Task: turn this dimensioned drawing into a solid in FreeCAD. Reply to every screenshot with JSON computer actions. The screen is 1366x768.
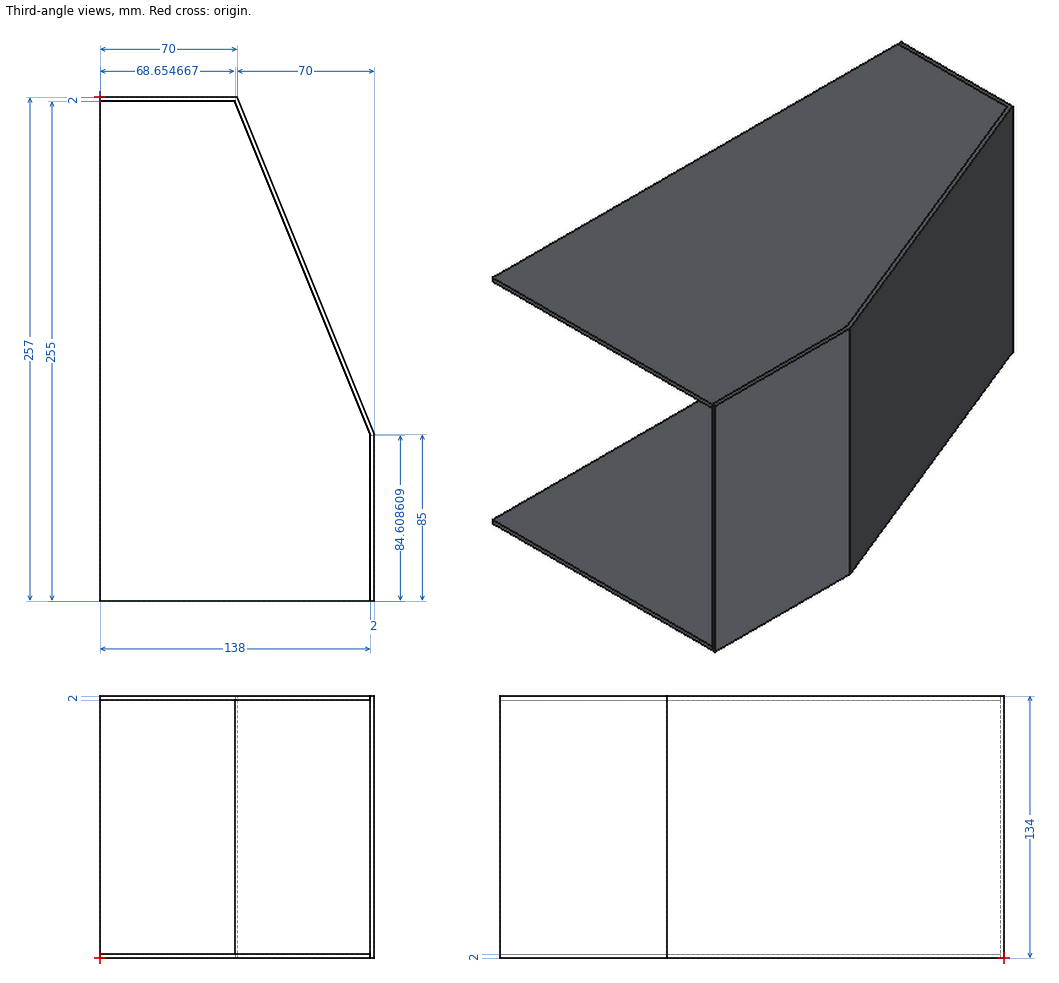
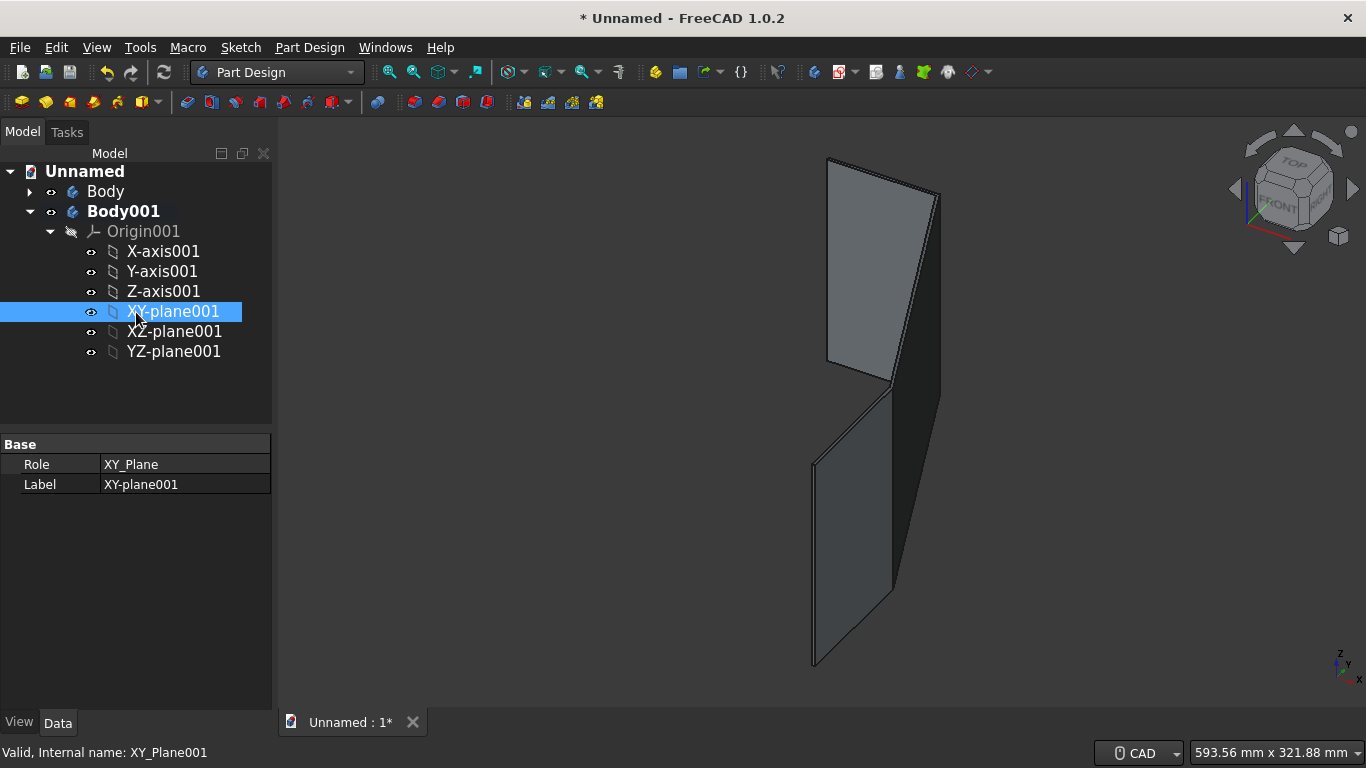
{"action": "left_click", "coordinate": [972, 72]}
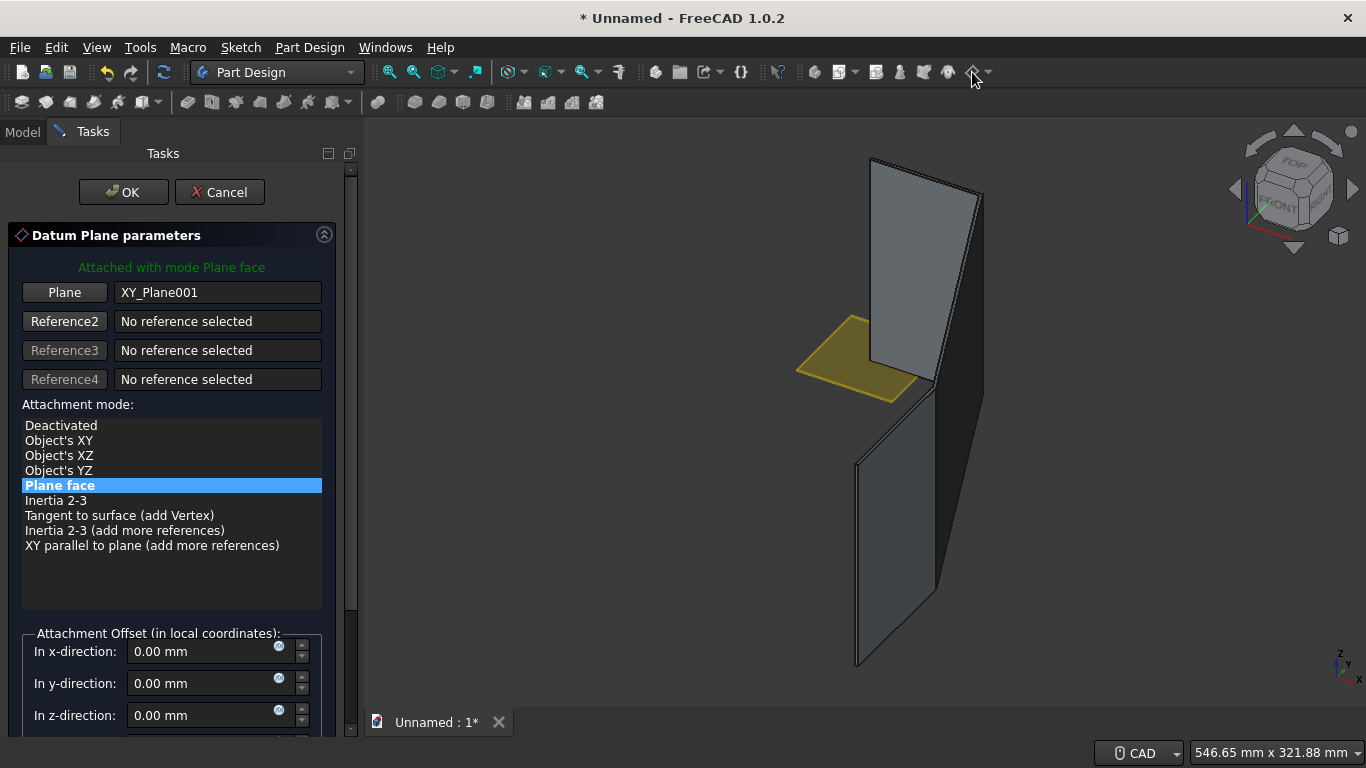
{"action": "triple_click", "coordinate": [210, 715]}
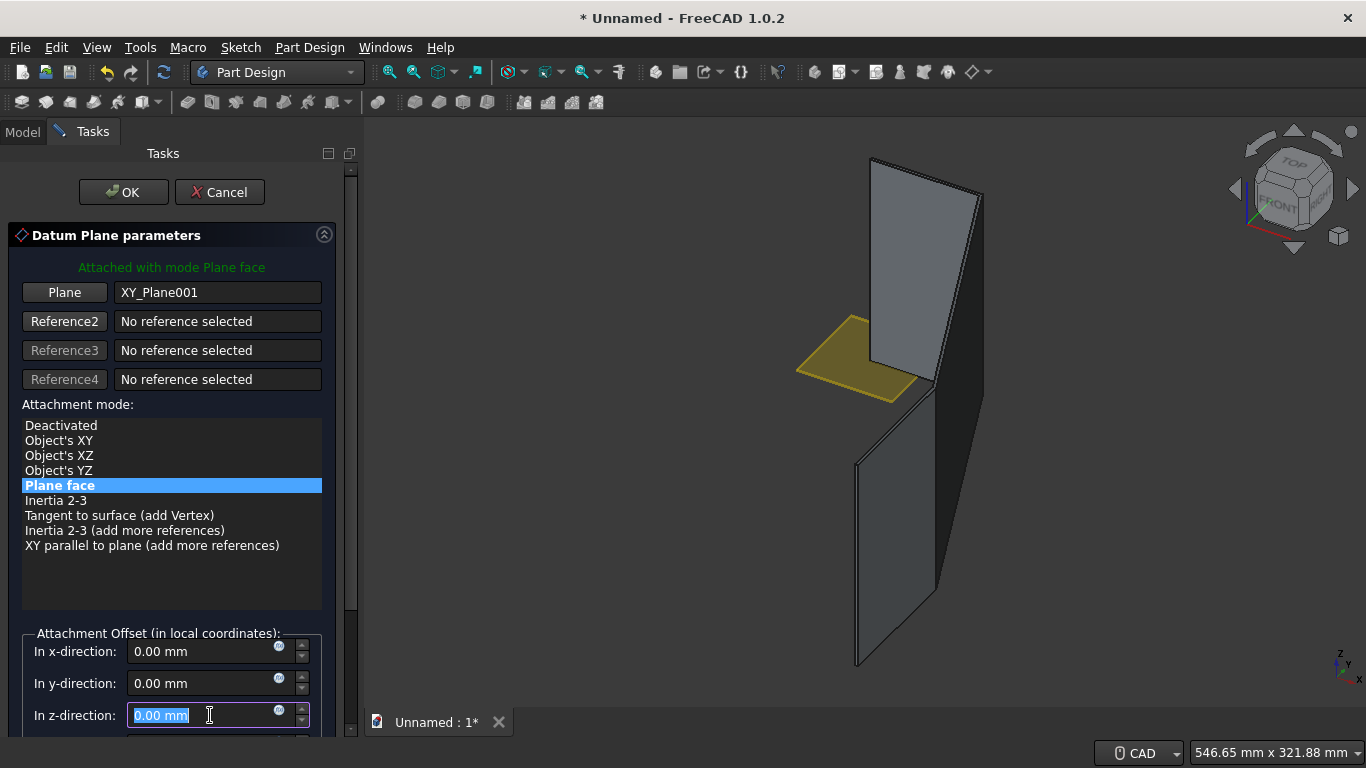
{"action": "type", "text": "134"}
{"action": "key", "text": "Tab"}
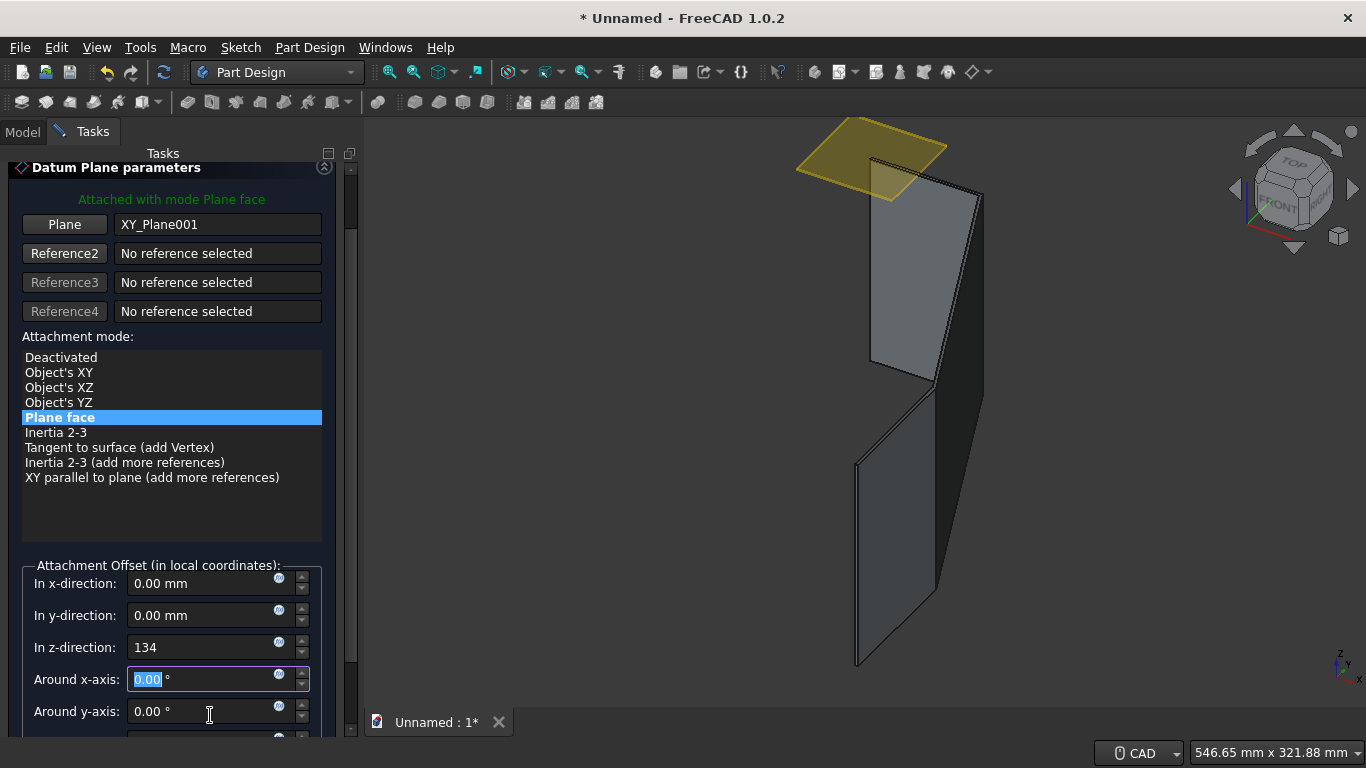
{"action": "scroll", "coordinate": [351, 450], "scroll_direction": "up", "scroll_amount": 2}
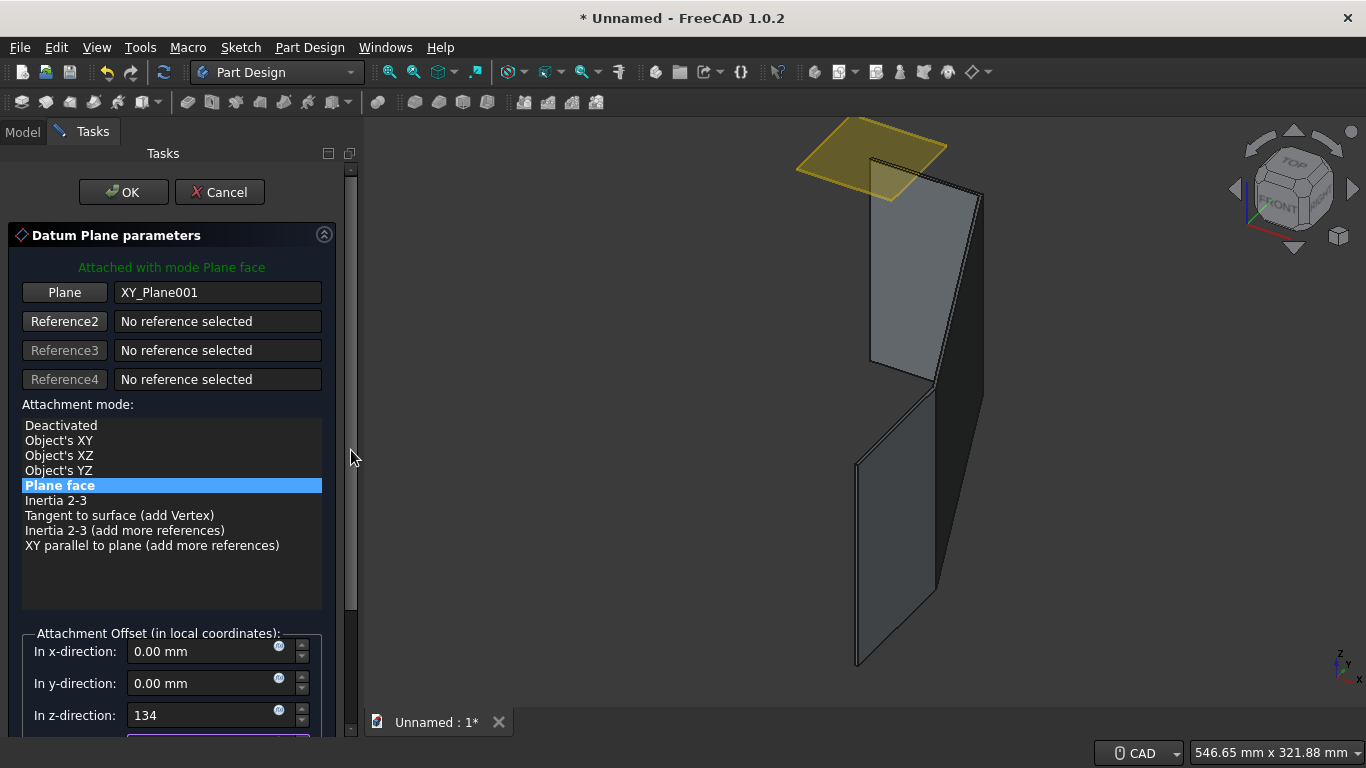
{"action": "left_click", "coordinate": [124, 192]}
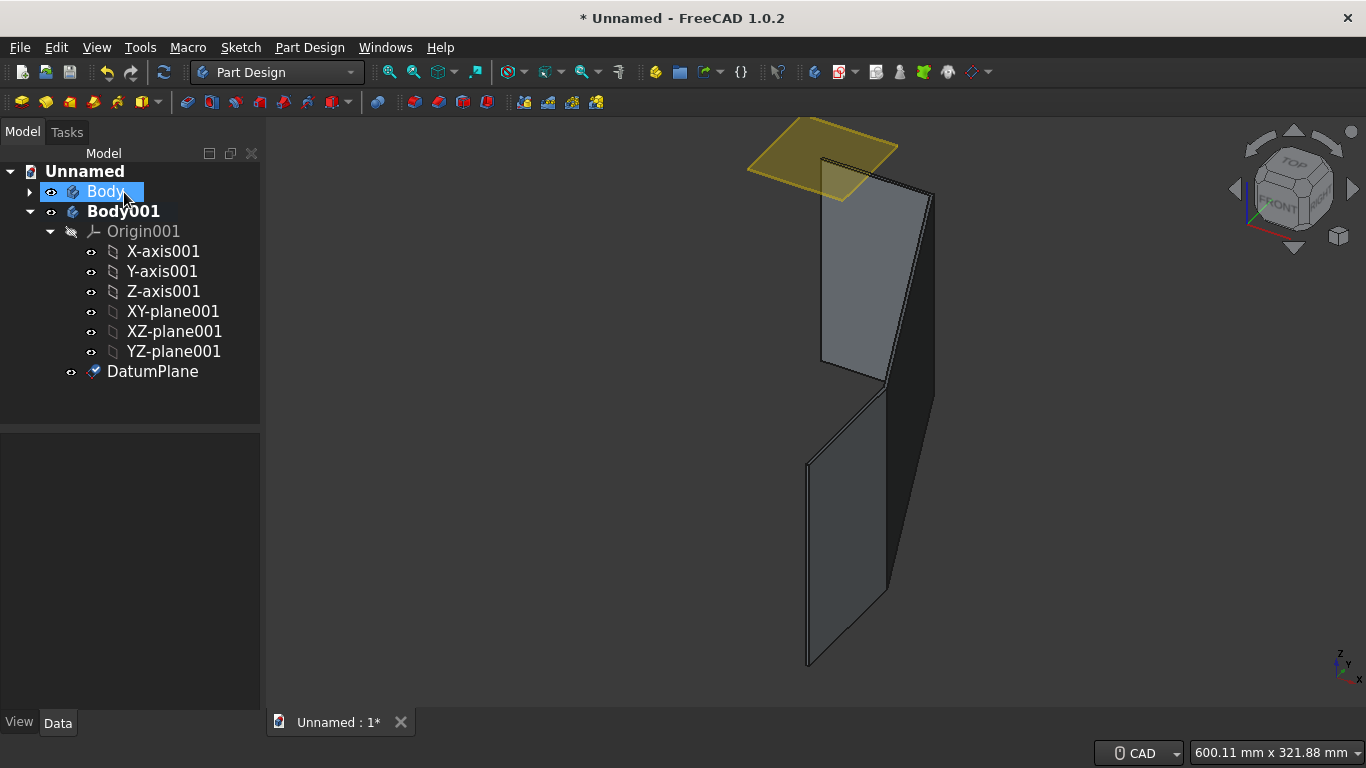
{"action": "left_click", "coordinate": [116, 372]}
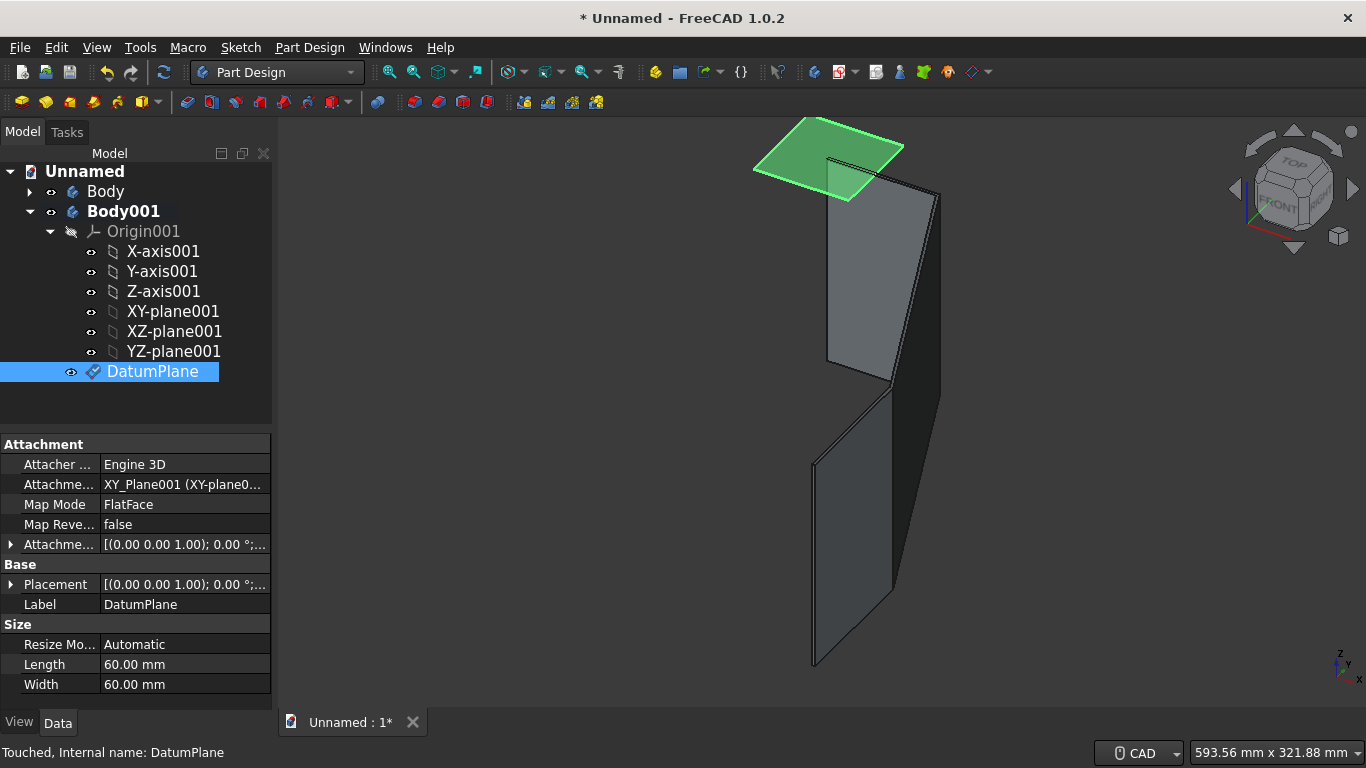
{"action": "left_click", "coordinate": [840, 72]}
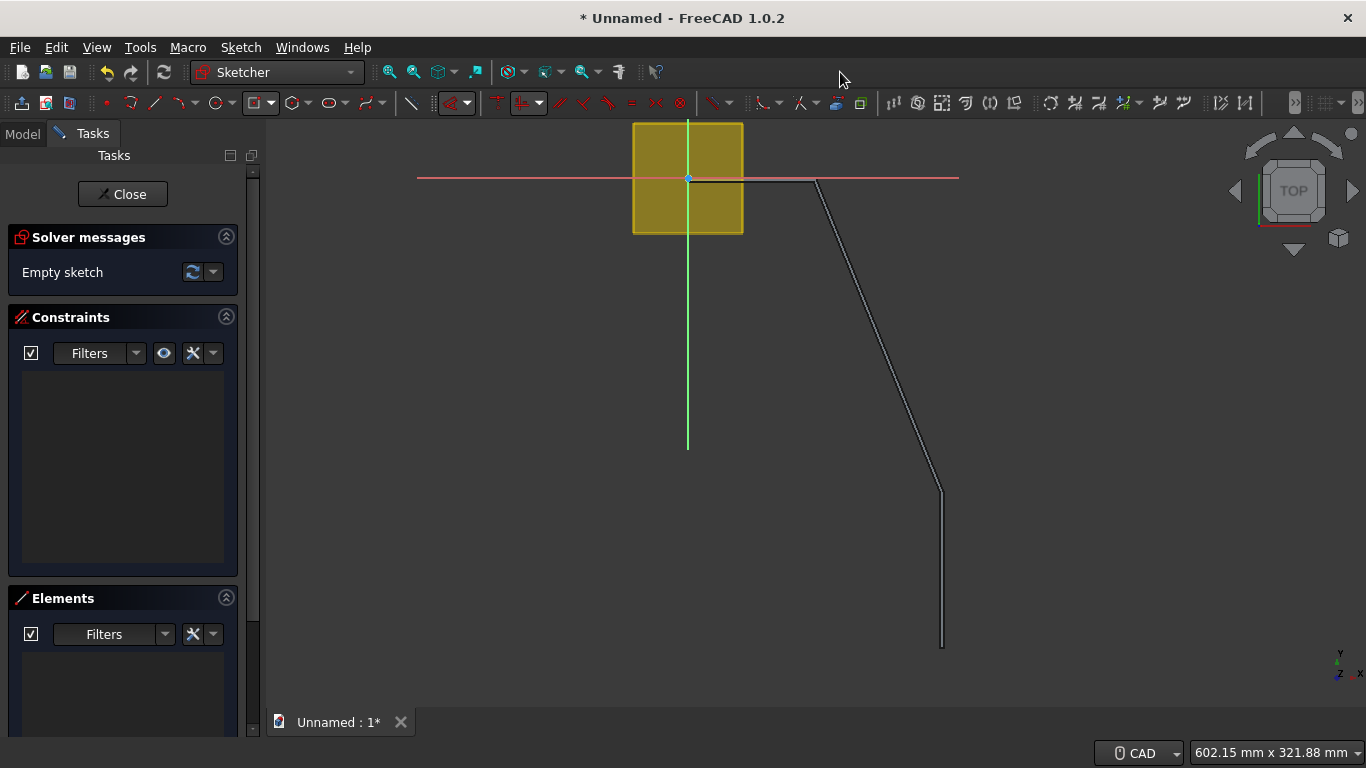
{"action": "key", "text": "g m"}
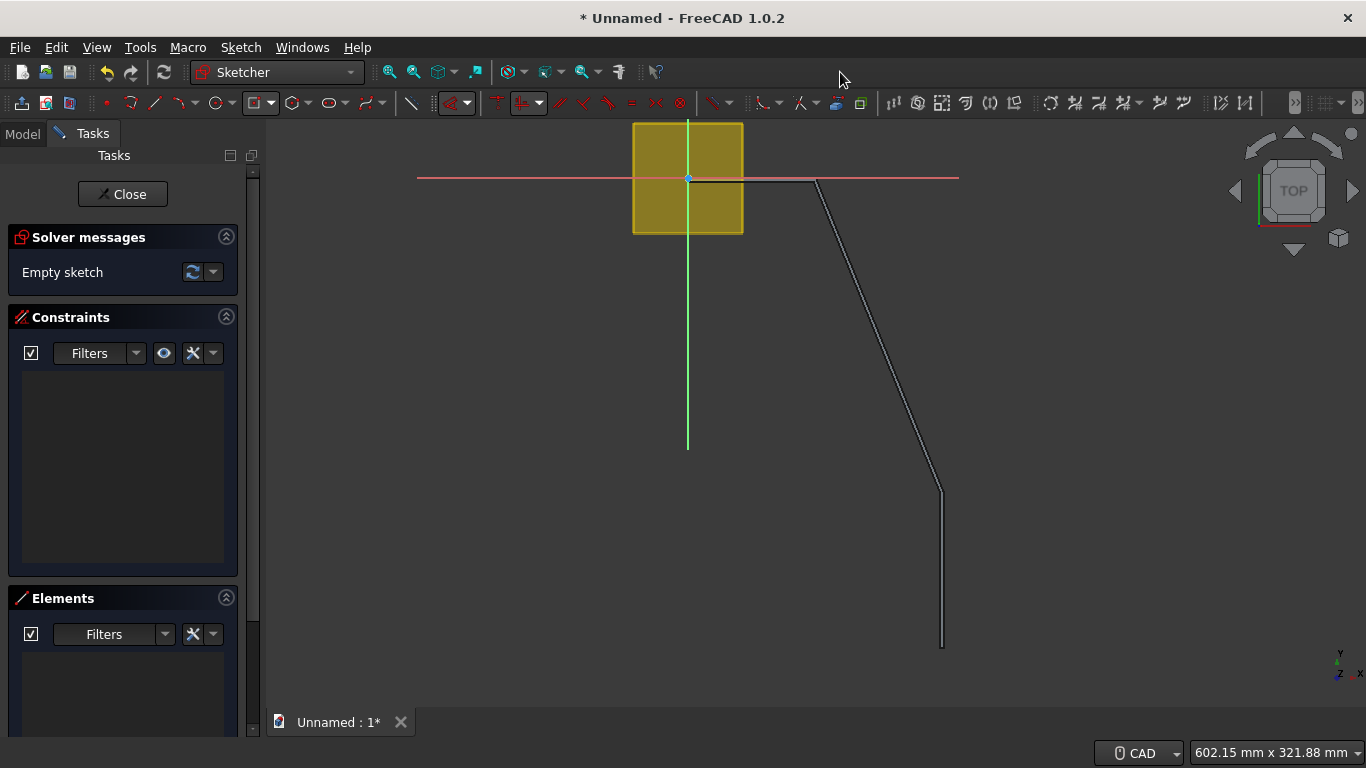
{"action": "scroll", "coordinate": [688, 182], "scroll_direction": "up", "scroll_amount": 8}